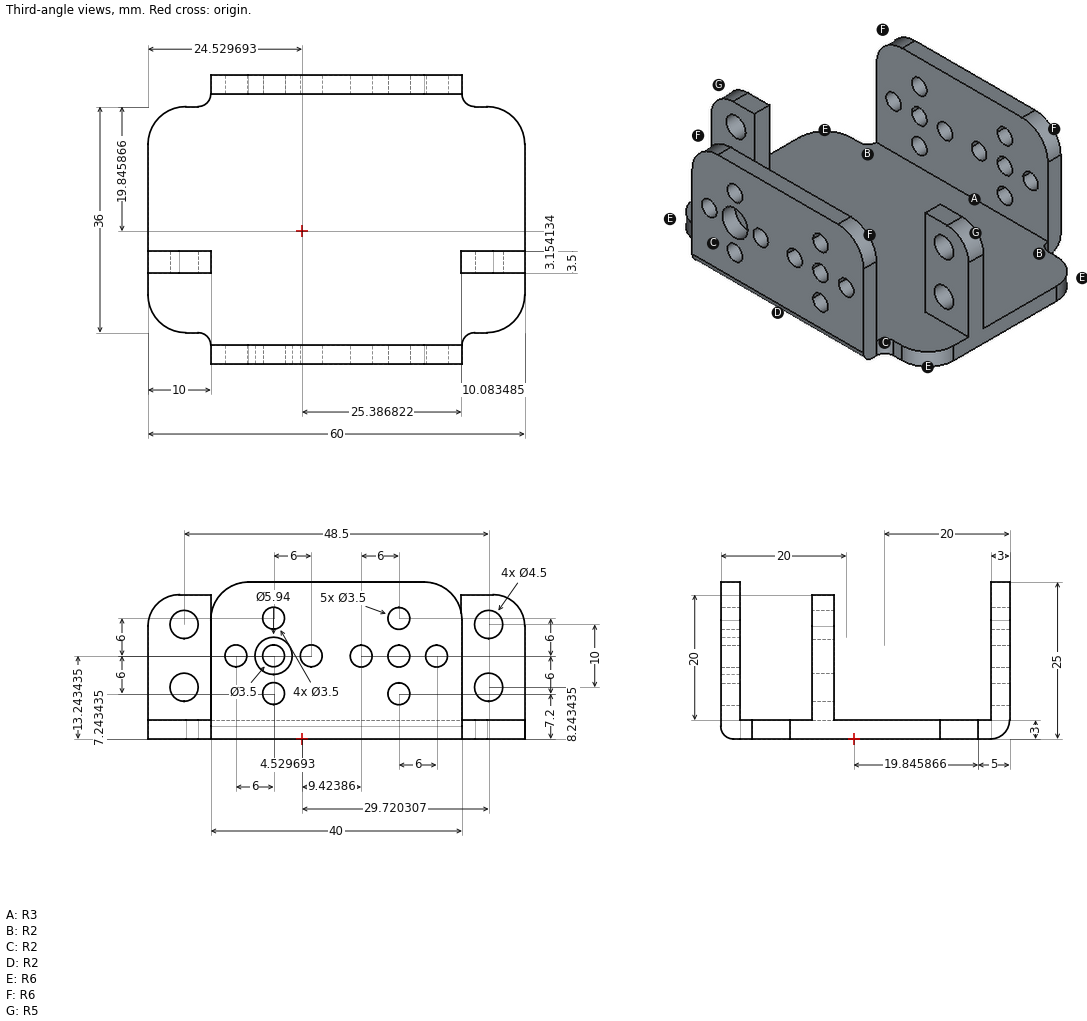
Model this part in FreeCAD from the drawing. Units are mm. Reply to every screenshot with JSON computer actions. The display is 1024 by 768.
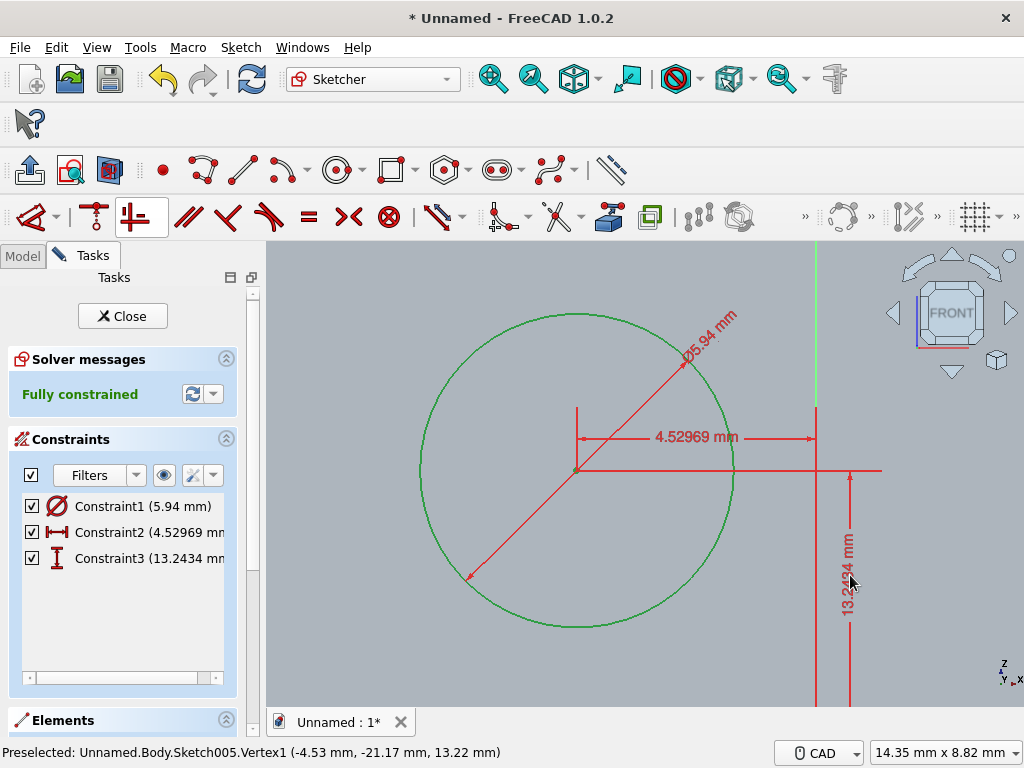
{"action": "left_click", "coordinate": [123, 316]}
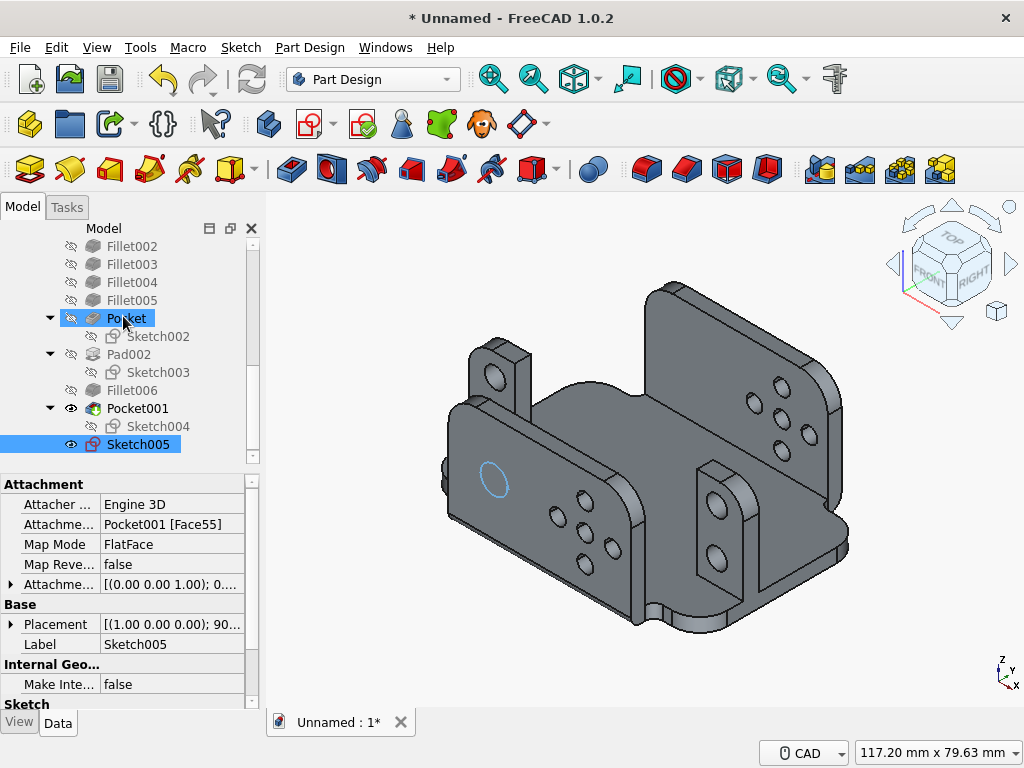
{"action": "left_click", "coordinate": [292, 170]}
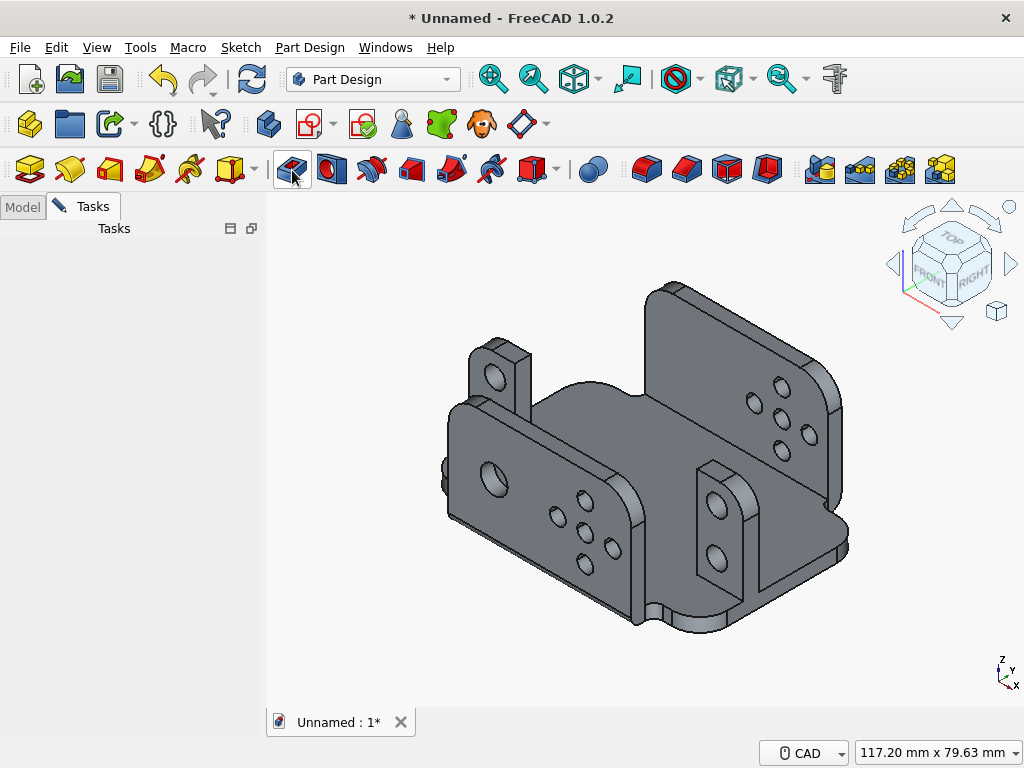
{"action": "type", "text": "20"}
{"action": "key", "text": "Tab"}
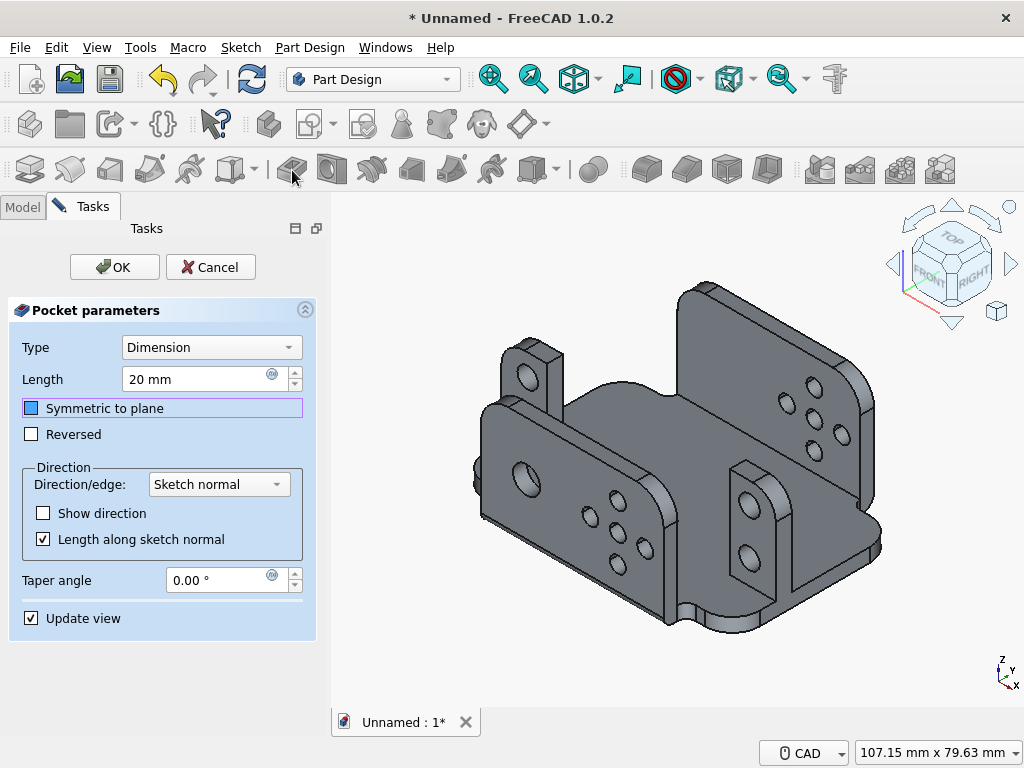
{"action": "left_click", "coordinate": [115, 267]}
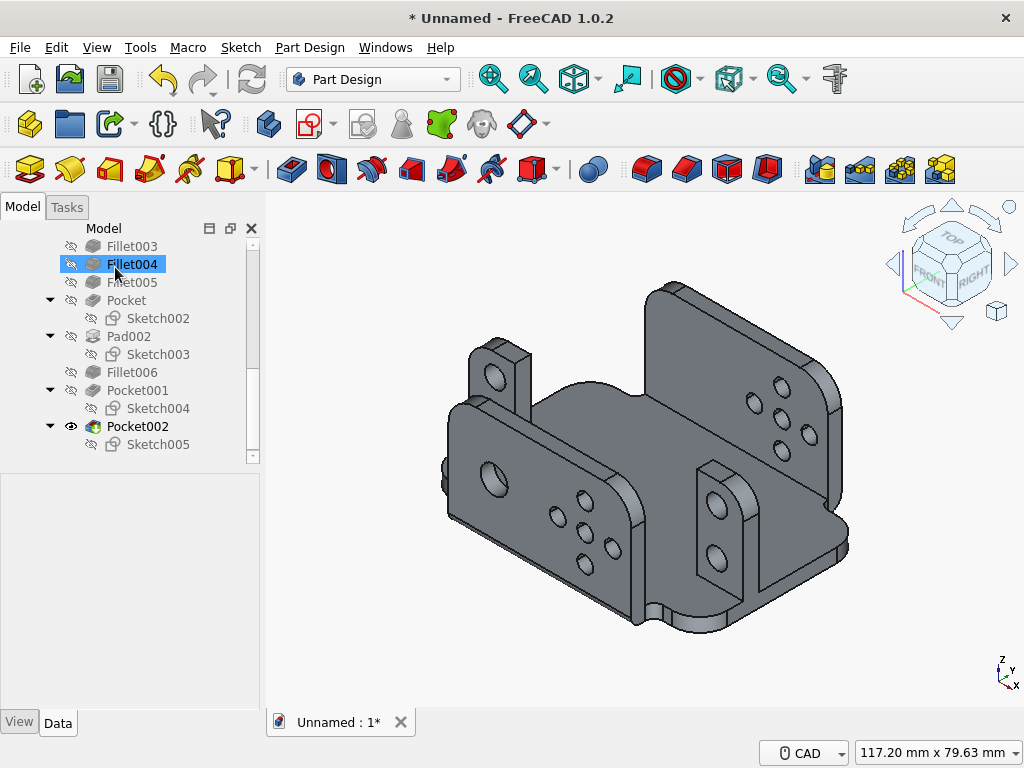
{"action": "left_click", "coordinate": [540, 469]}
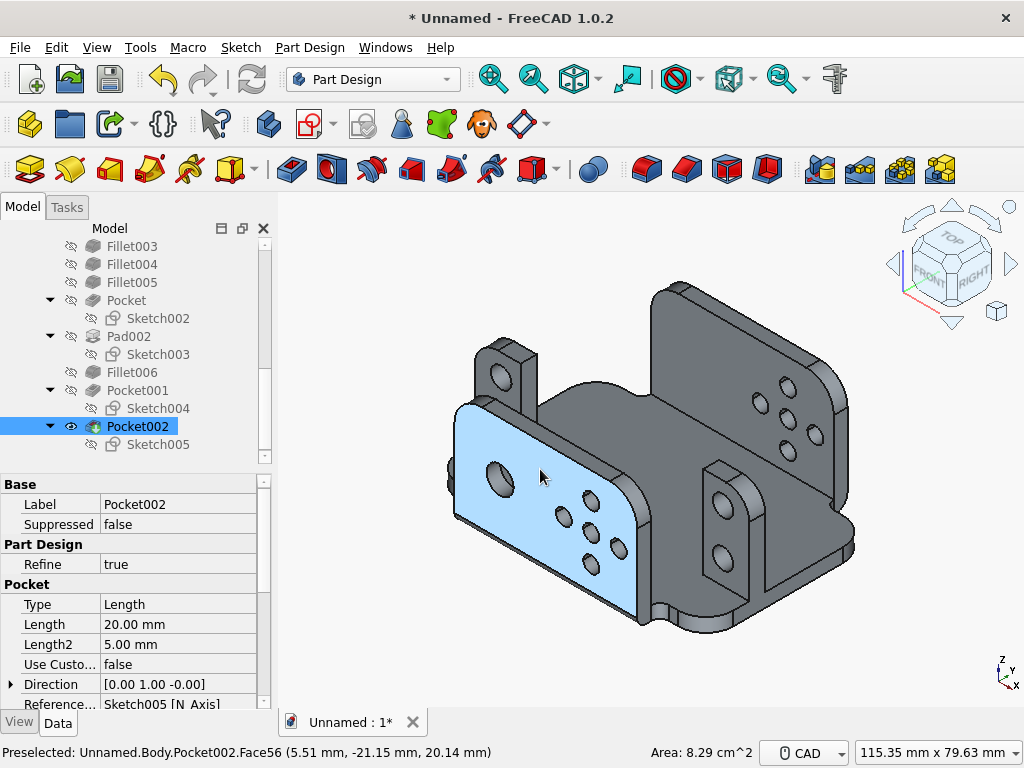
{"action": "left_click", "coordinate": [310, 124]}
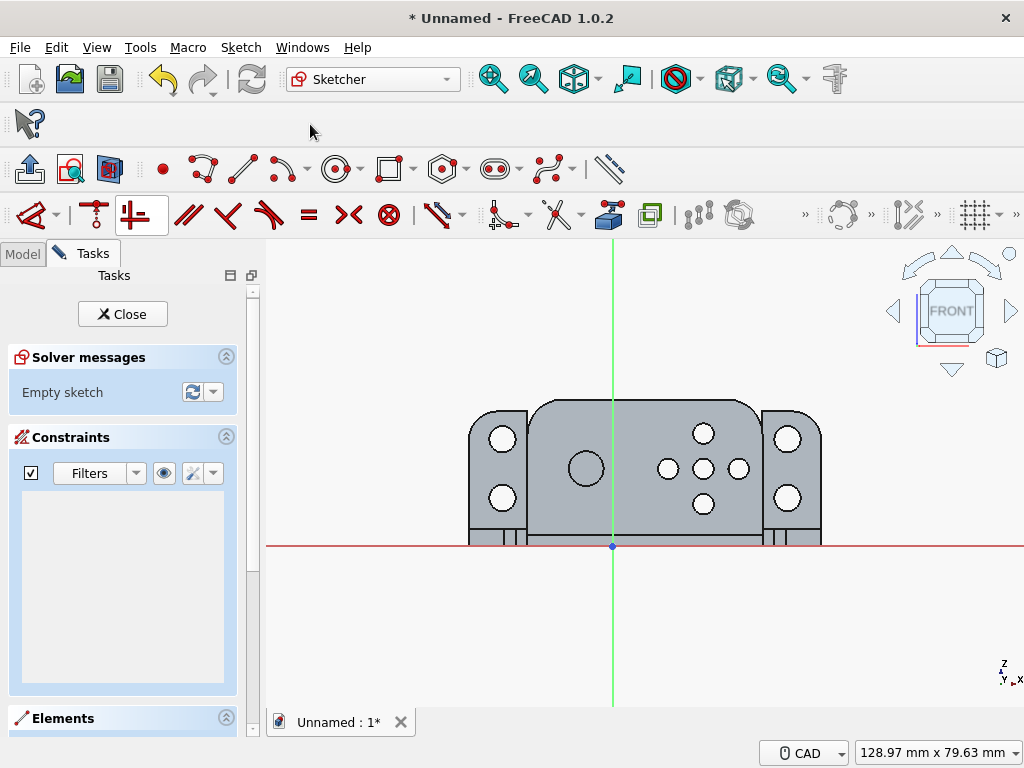
{"action": "scroll", "coordinate": [594, 494], "scroll_direction": "up", "scroll_amount": 4}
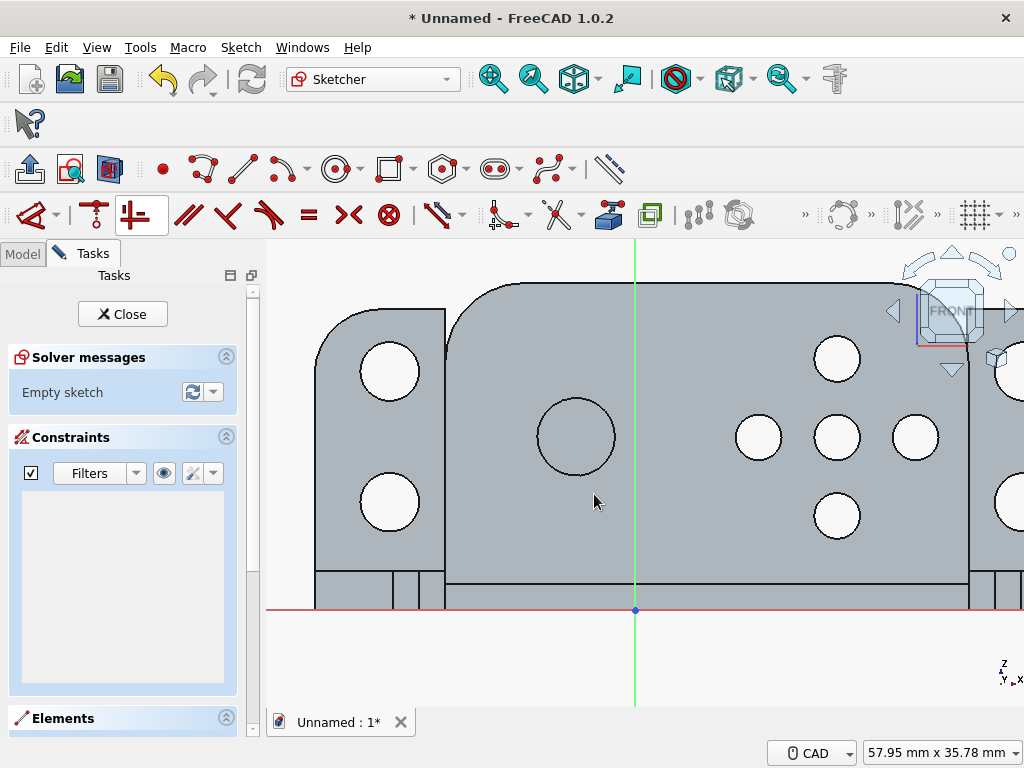
{"action": "left_click", "coordinate": [336, 170]}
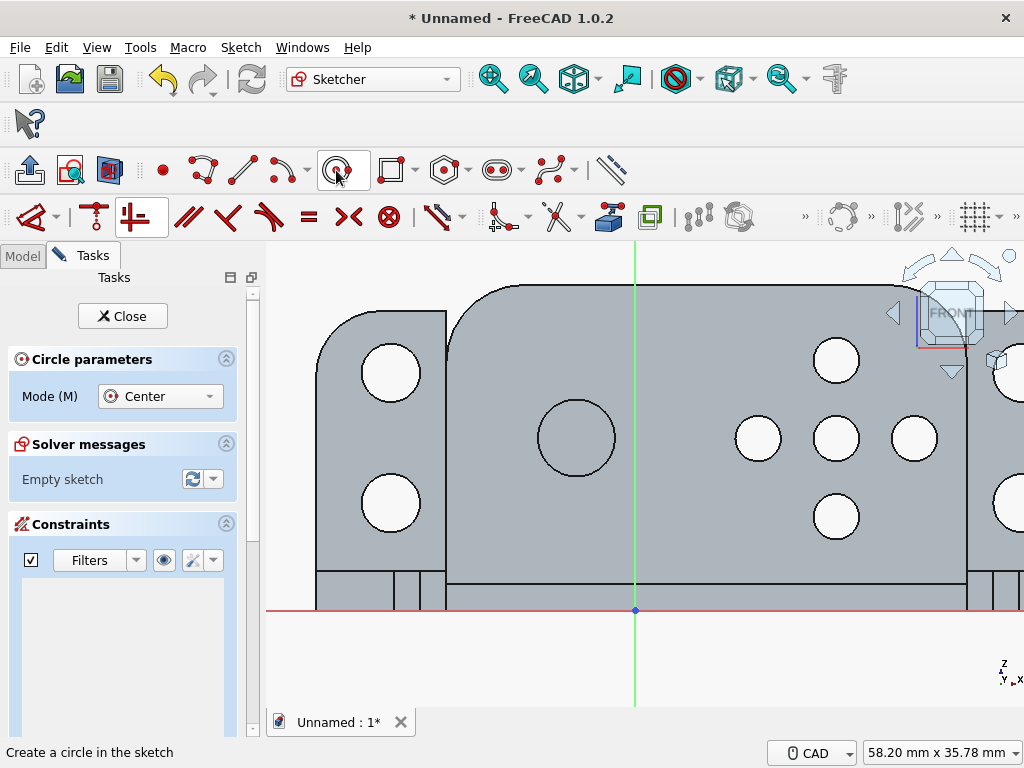
{"action": "left_click", "coordinate": [576, 360]}
{"action": "left_click", "coordinate": [593, 344]}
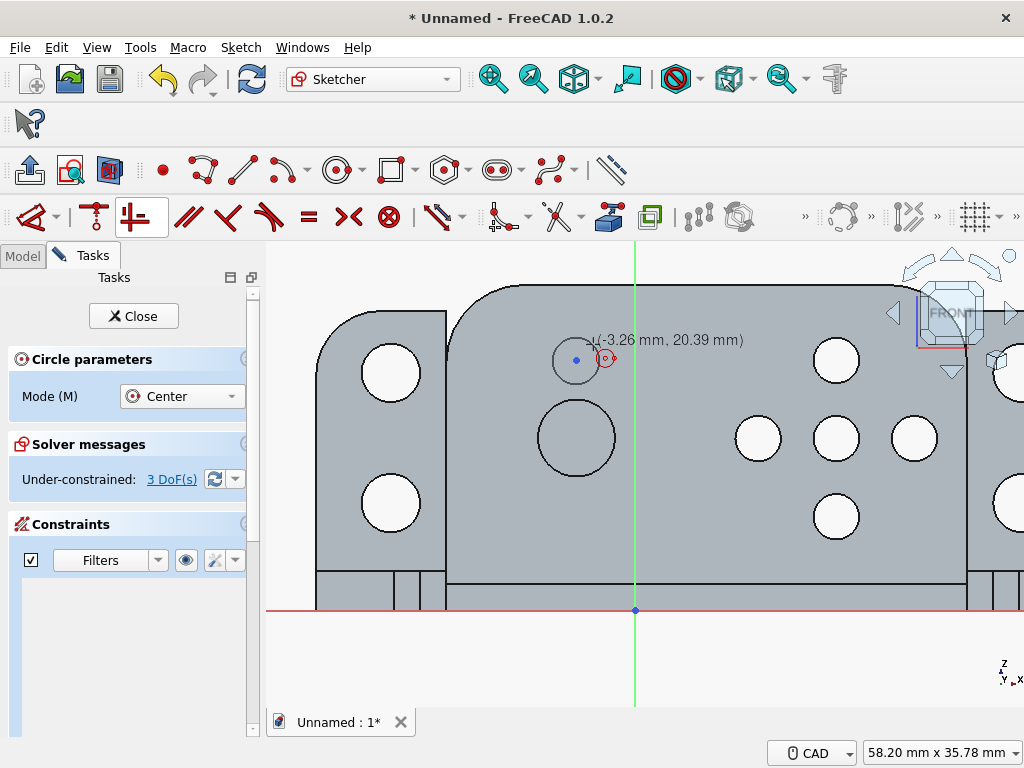
{"action": "left_click", "coordinate": [655, 438]}
{"action": "left_click", "coordinate": [671, 422]}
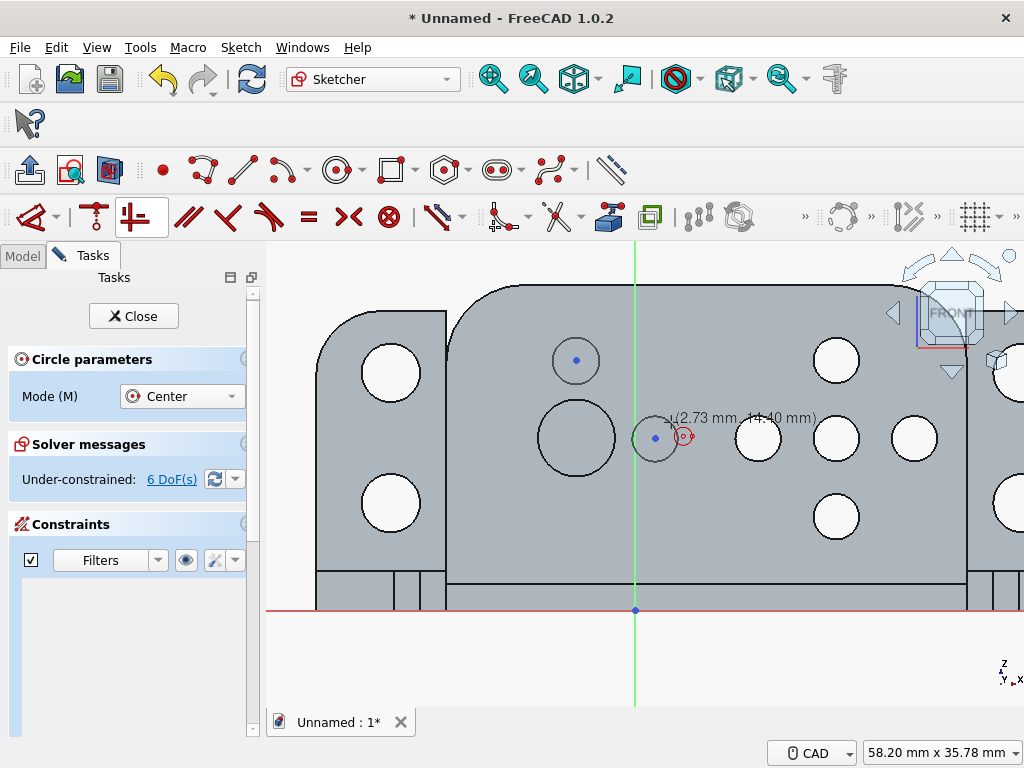
{"action": "left_click", "coordinate": [576, 516]}
{"action": "left_click", "coordinate": [593, 500]}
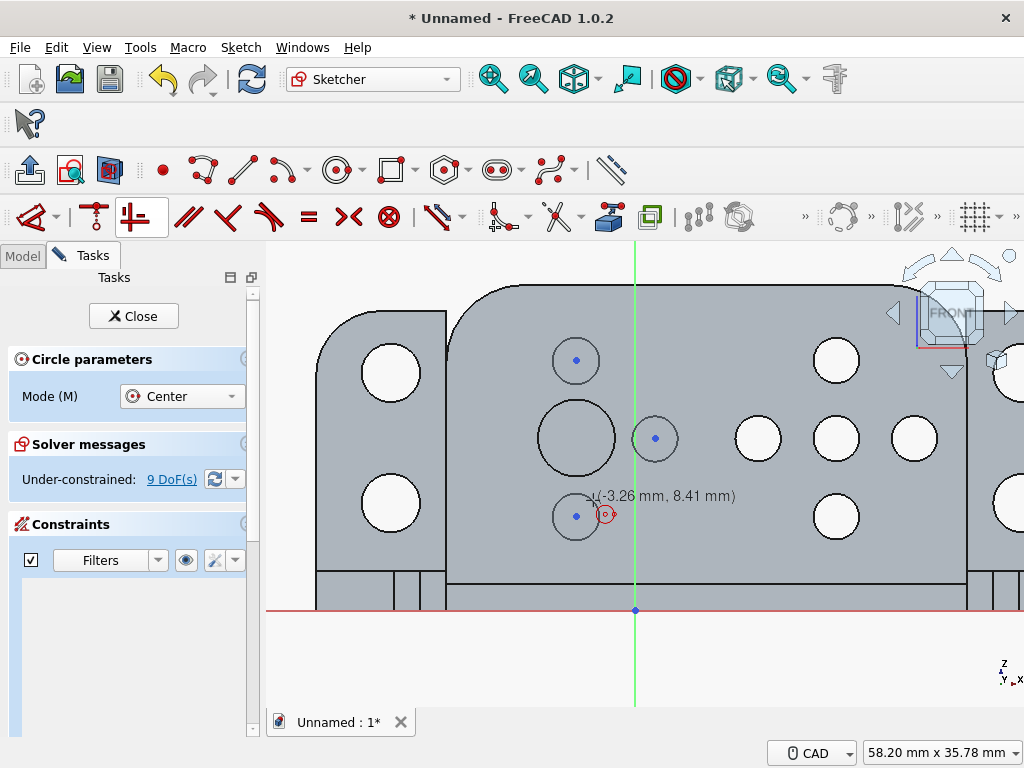
{"action": "left_click", "coordinate": [498, 438]}
{"action": "left_click", "coordinate": [514, 422]}
{"action": "key", "text": "Escape"}